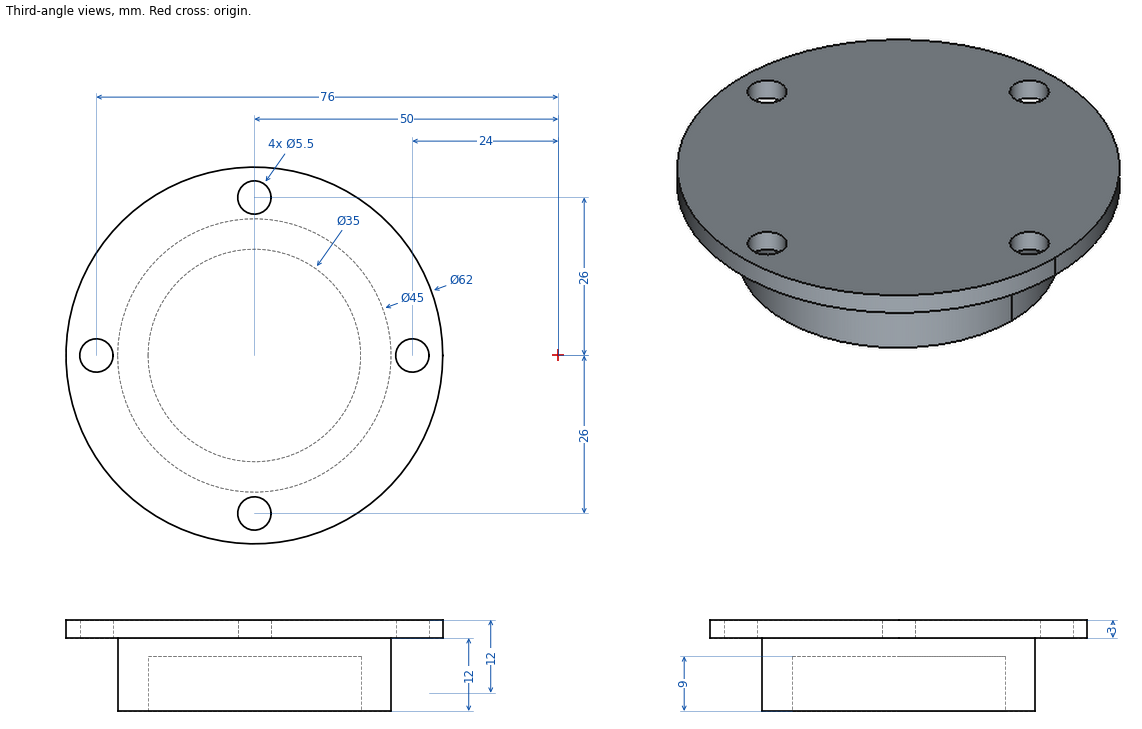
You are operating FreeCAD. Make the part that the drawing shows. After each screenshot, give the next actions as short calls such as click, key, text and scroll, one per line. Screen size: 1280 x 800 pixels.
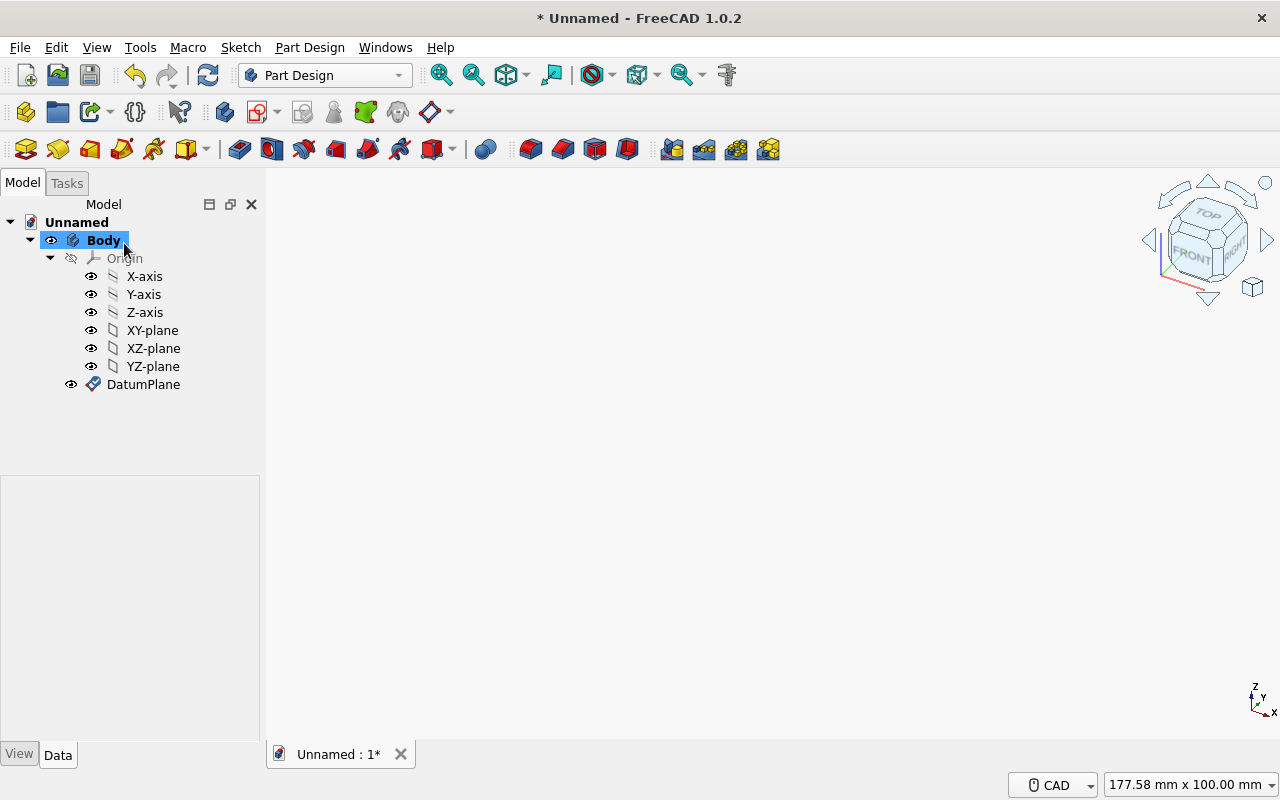
click(116, 384)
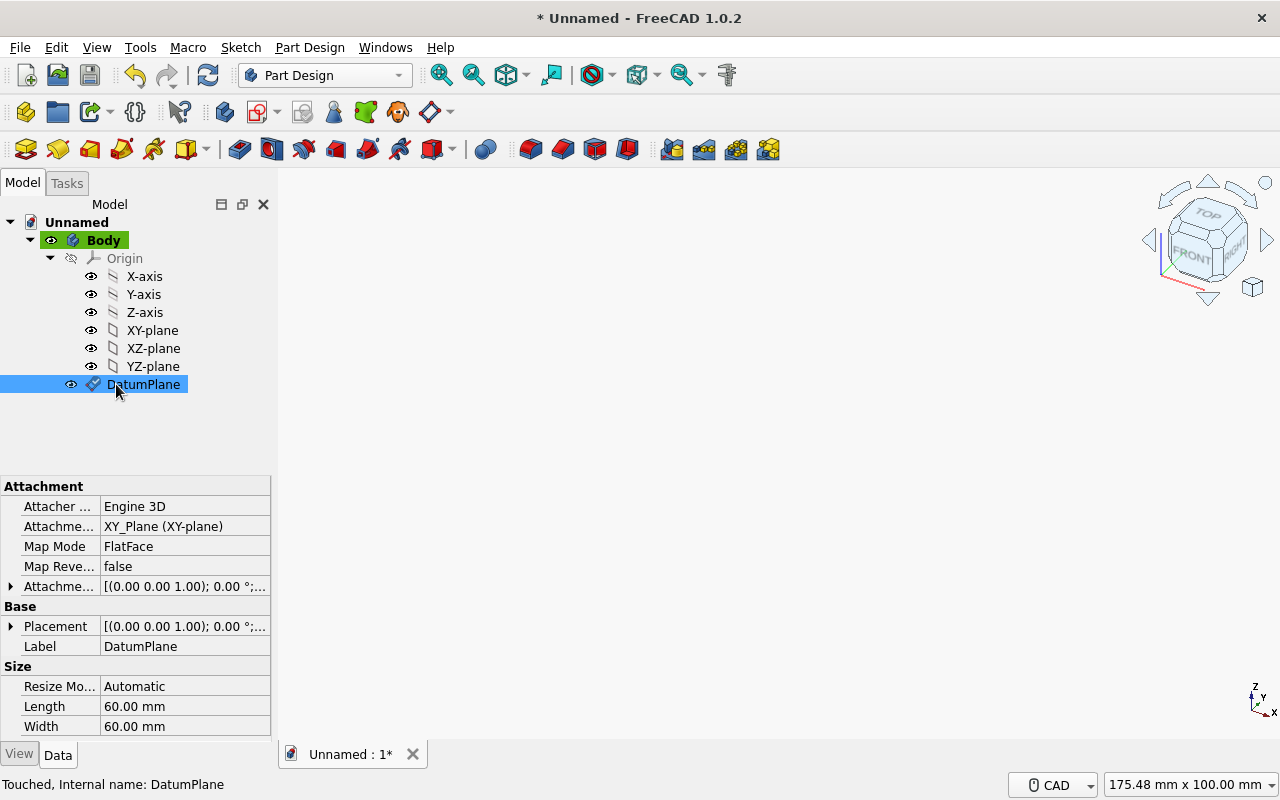
click(258, 112)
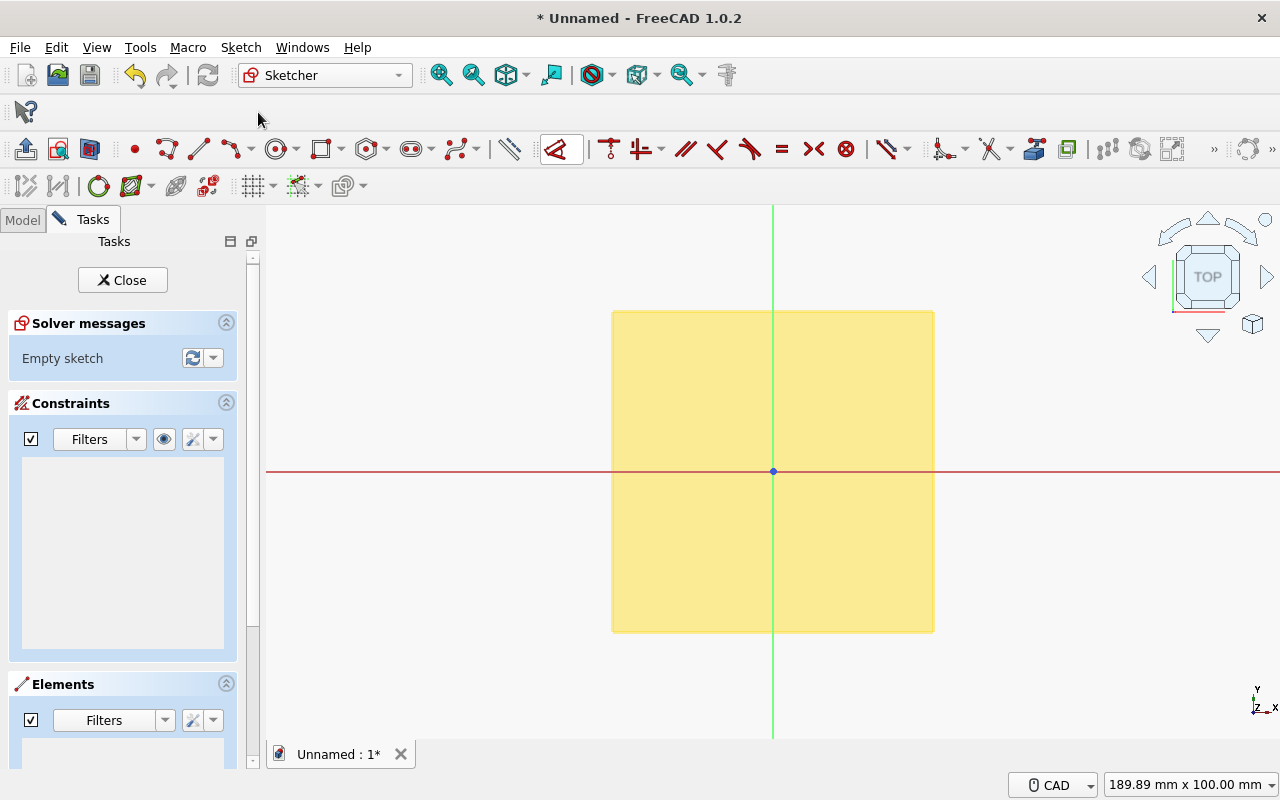
click(276, 150)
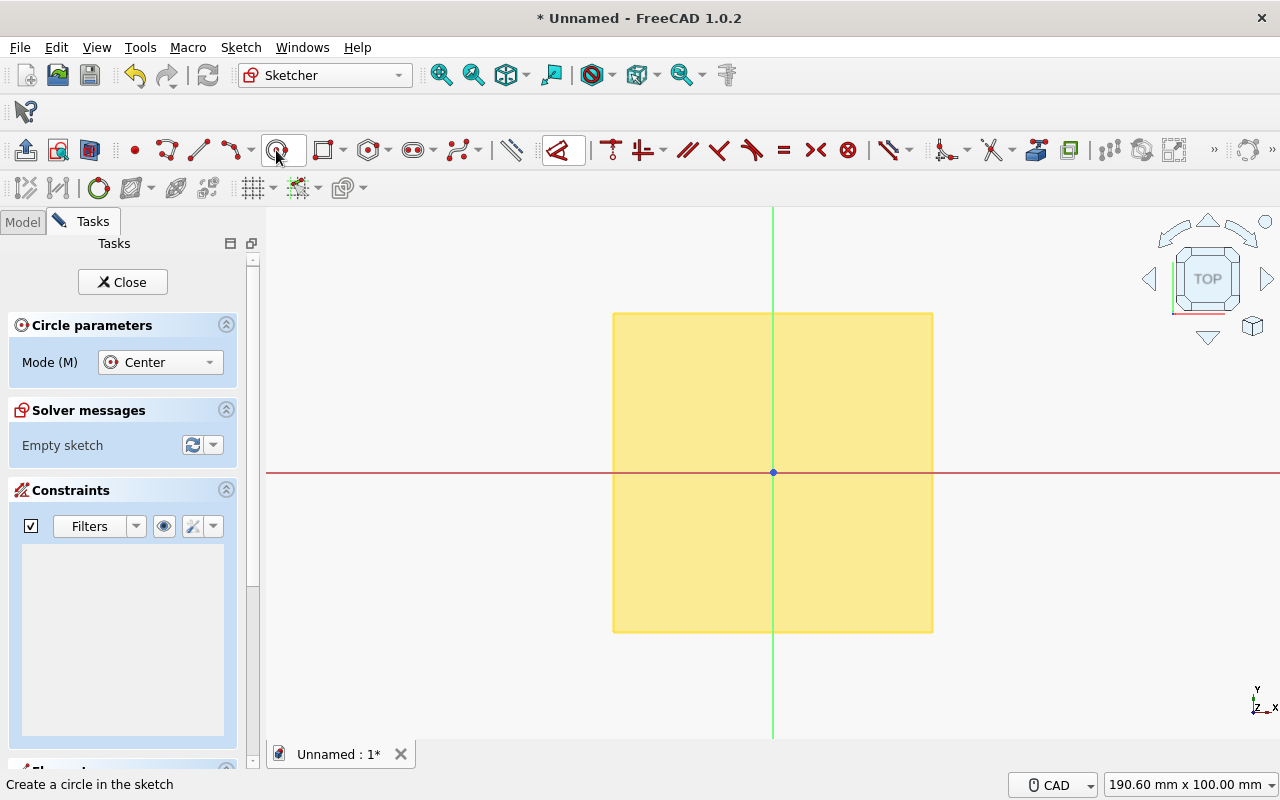
click(507, 473)
move(624, 356)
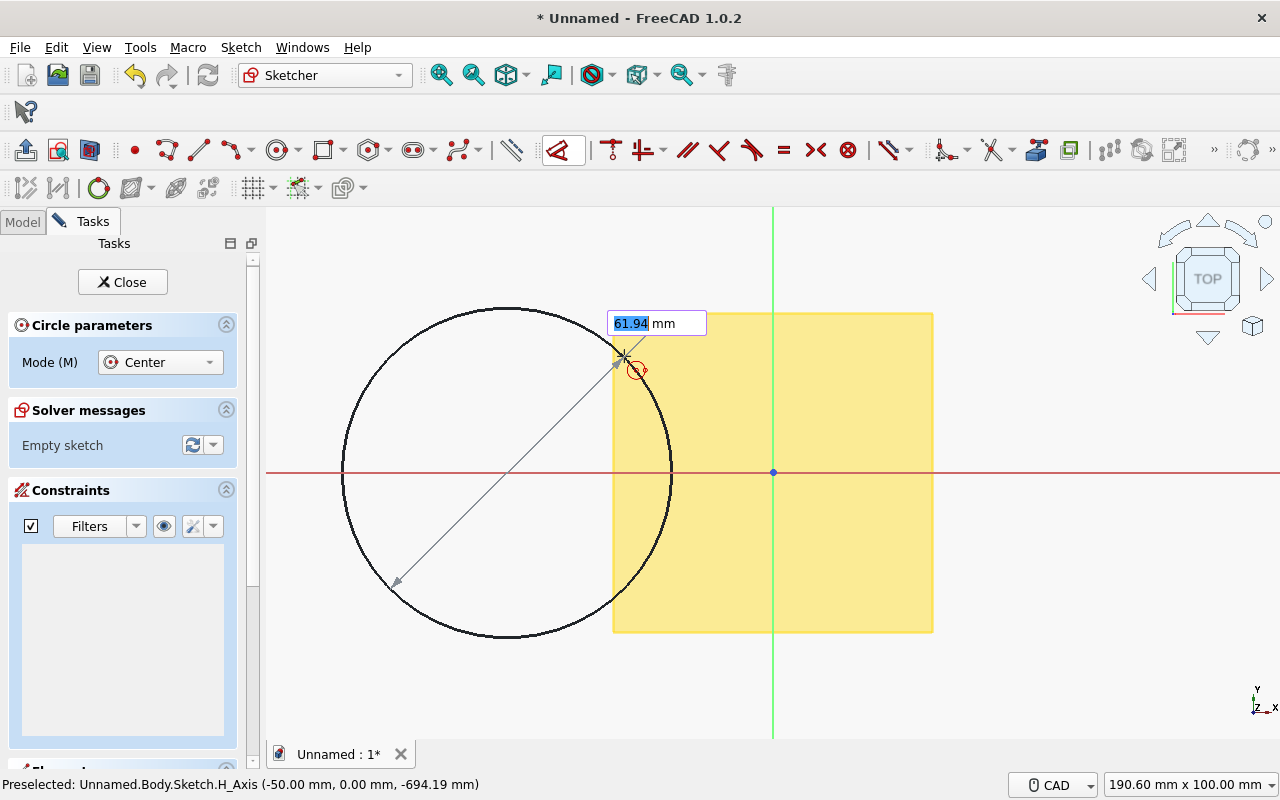
text(62)
key(Return)
key(Escape)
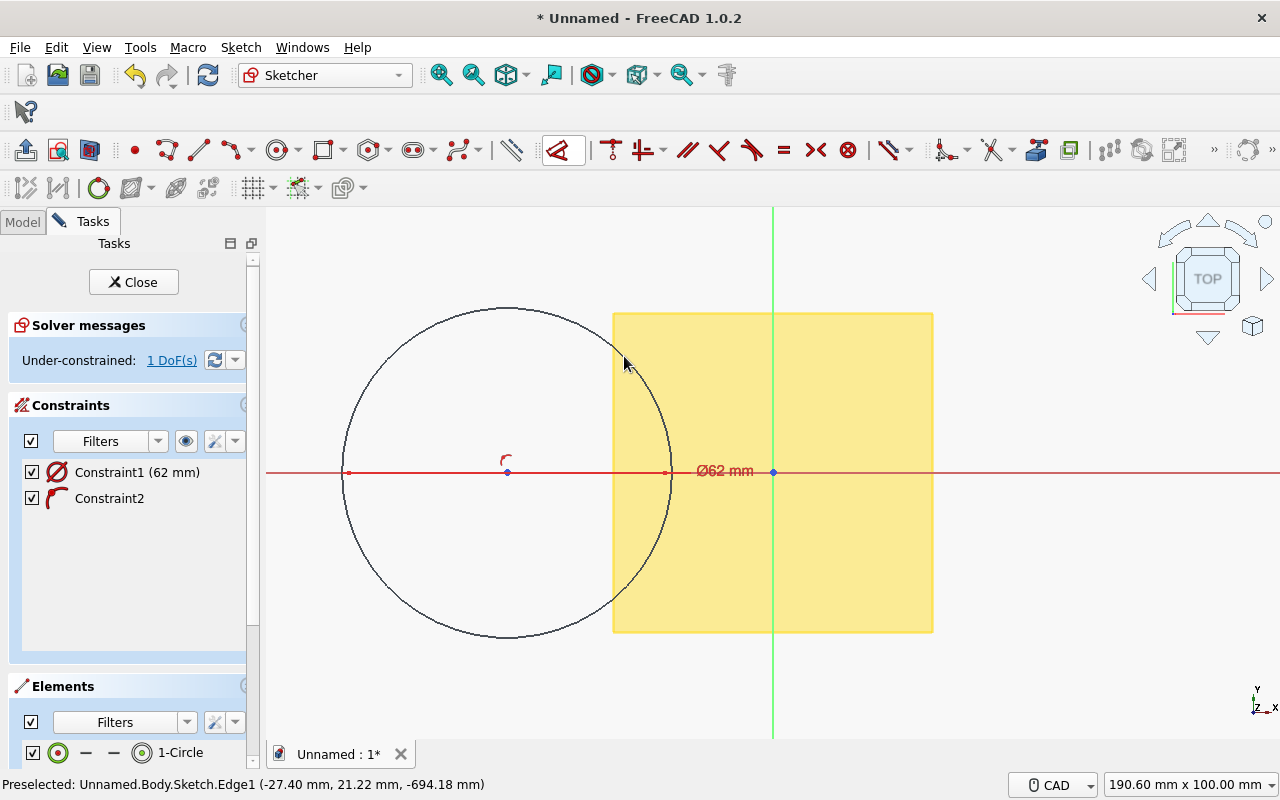
click(558, 150)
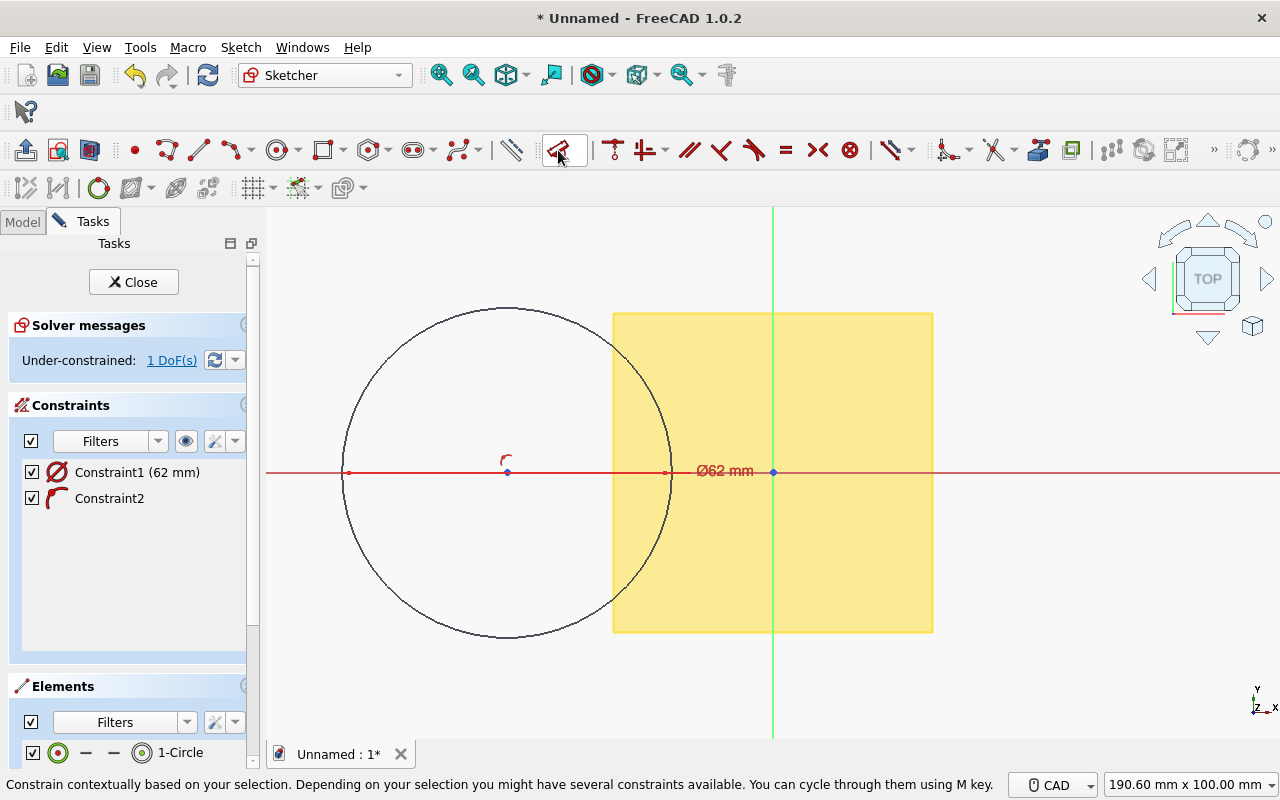
click(507, 473)
click(640, 507)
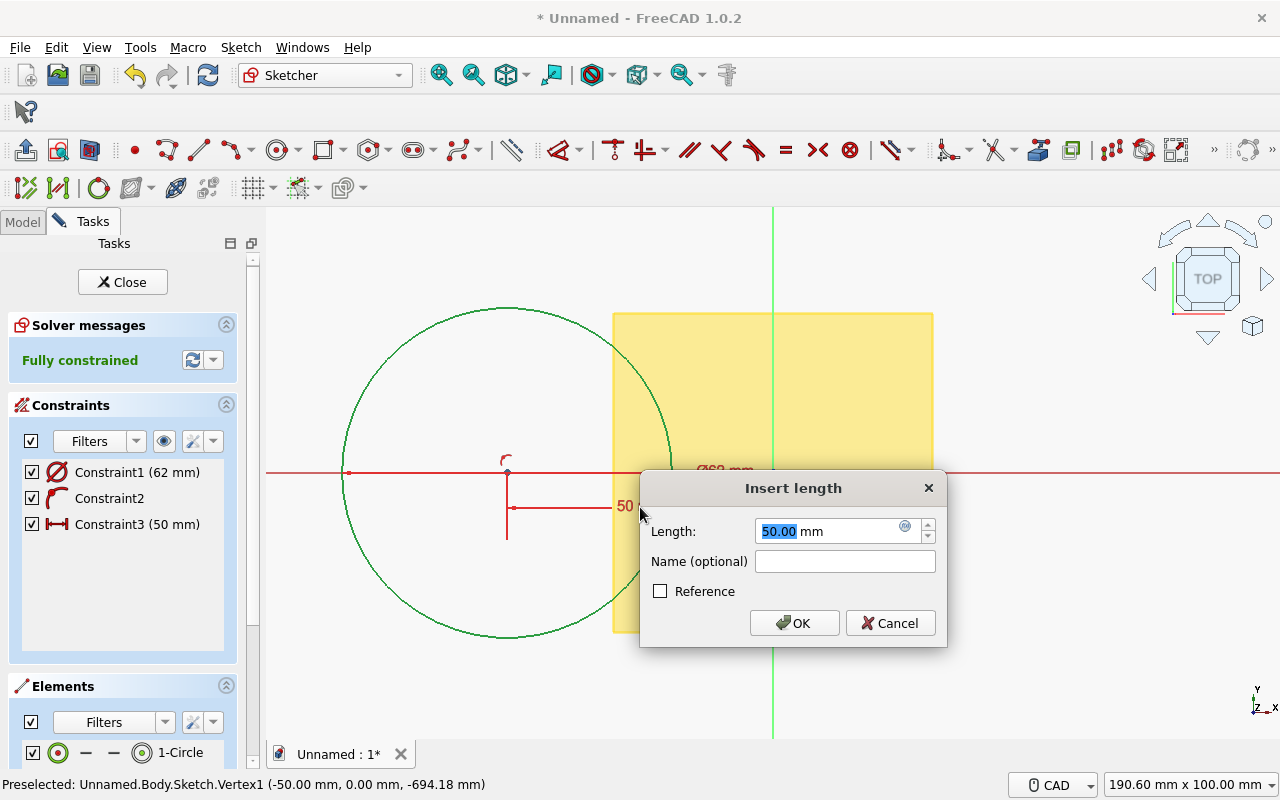
text(50)
key(Return)
key(Escape)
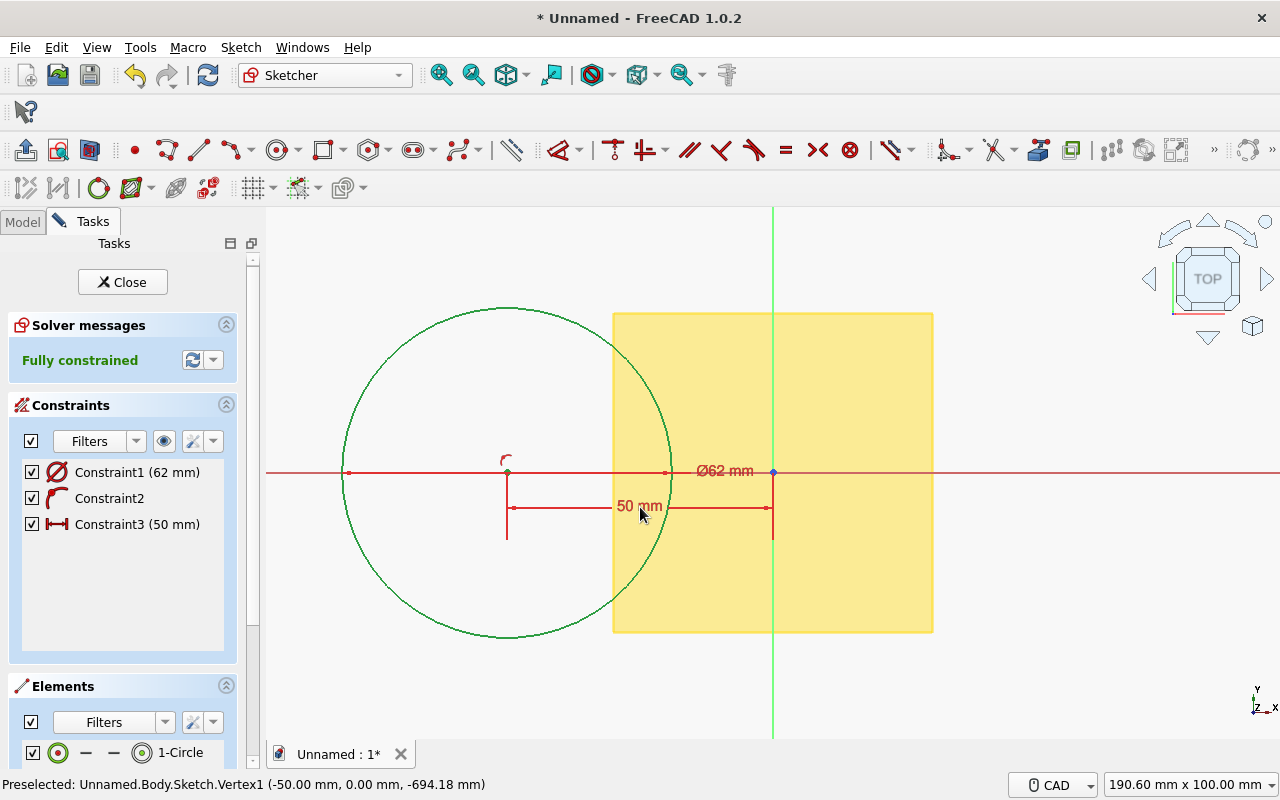
click(123, 282)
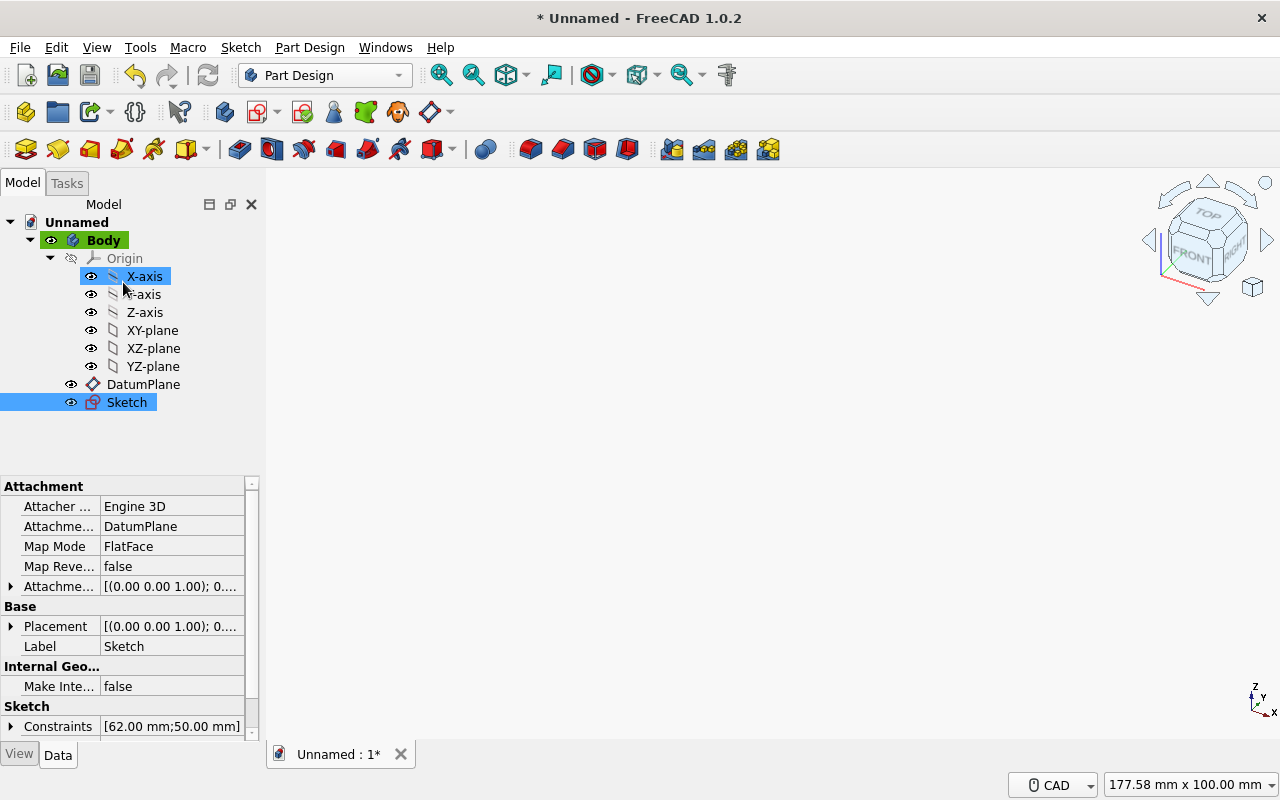
click(26, 150)